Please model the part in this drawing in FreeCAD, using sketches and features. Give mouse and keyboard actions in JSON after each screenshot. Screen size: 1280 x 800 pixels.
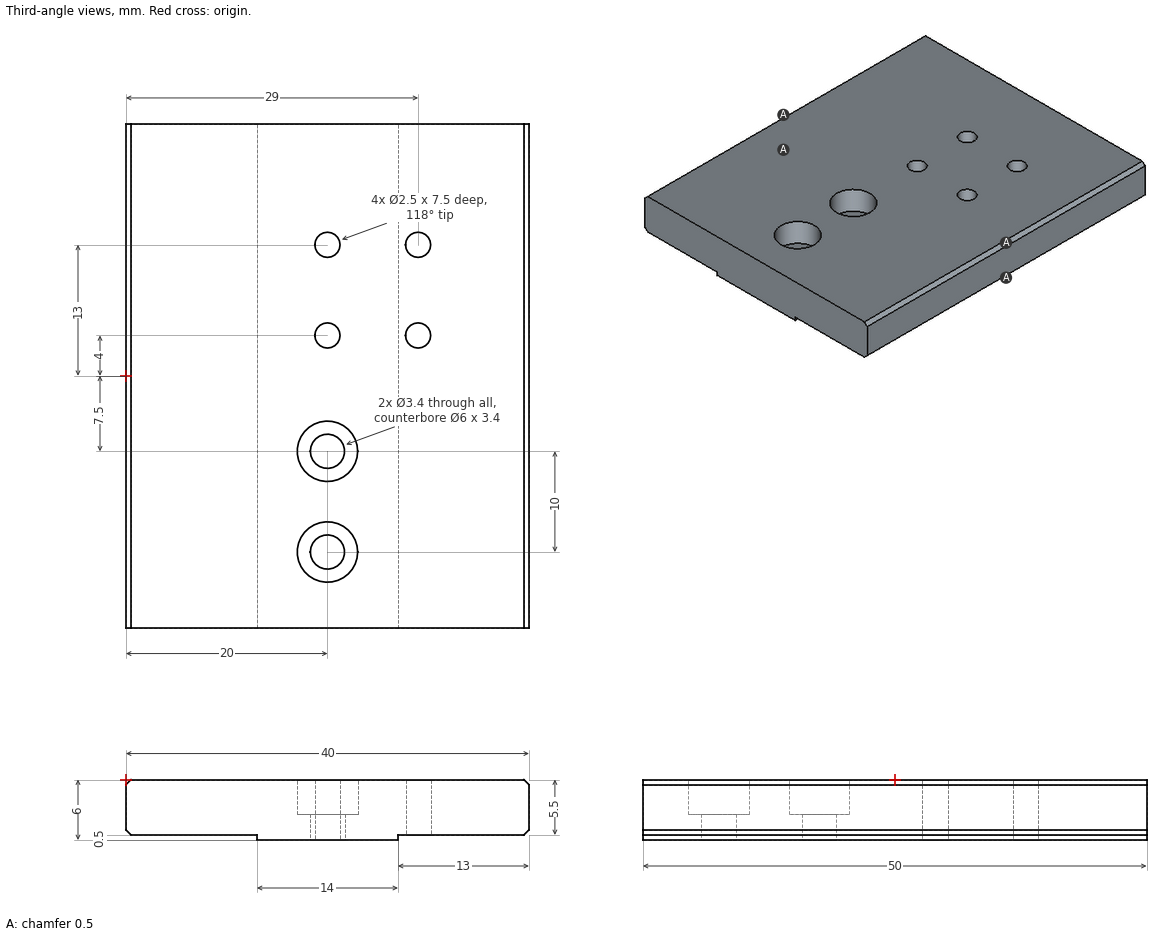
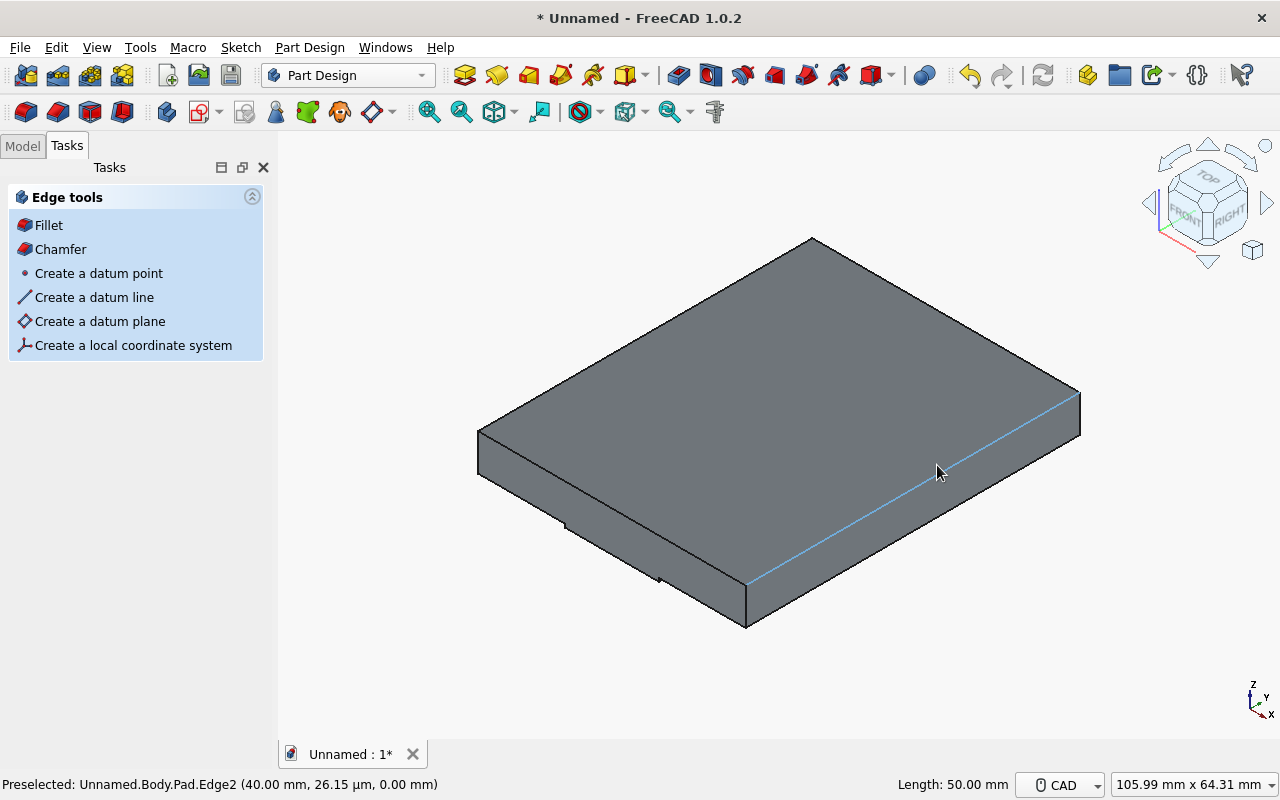
{"action": "key", "text": "2"}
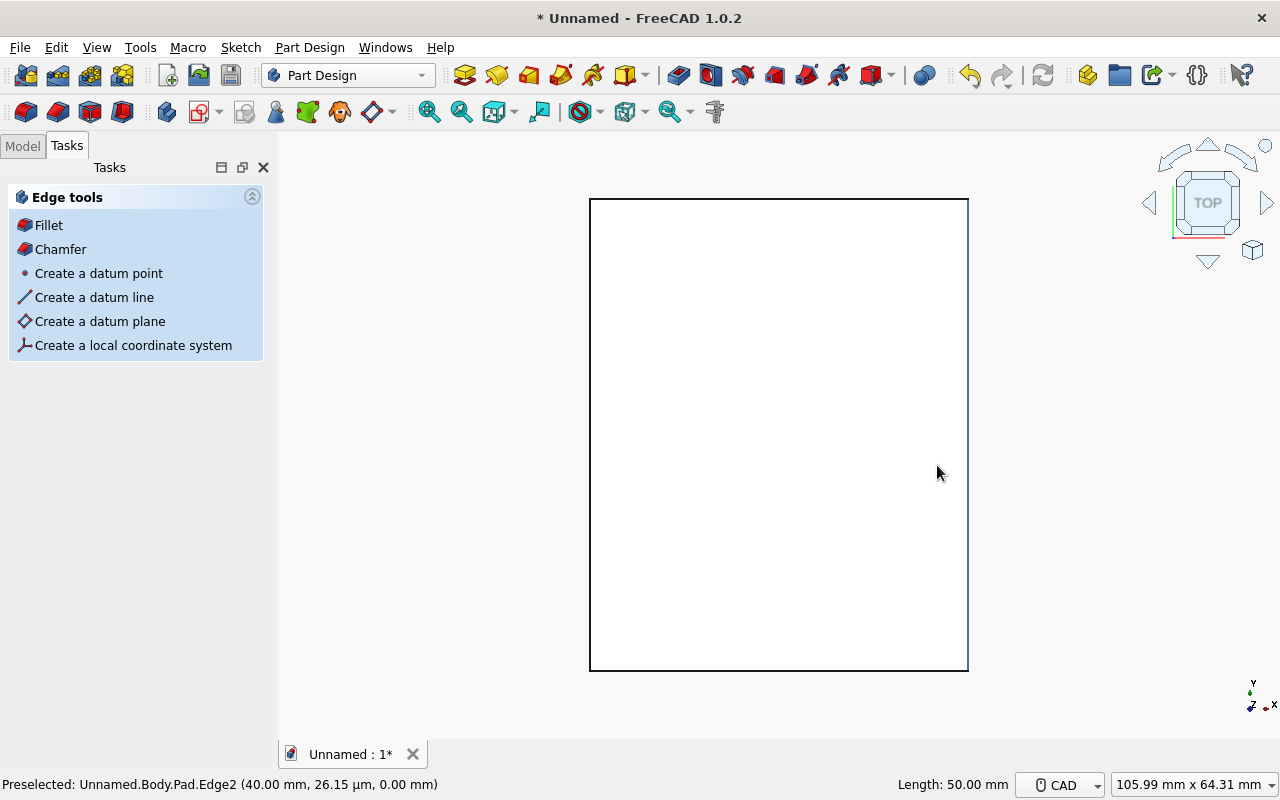
{"action": "key", "text": "1"}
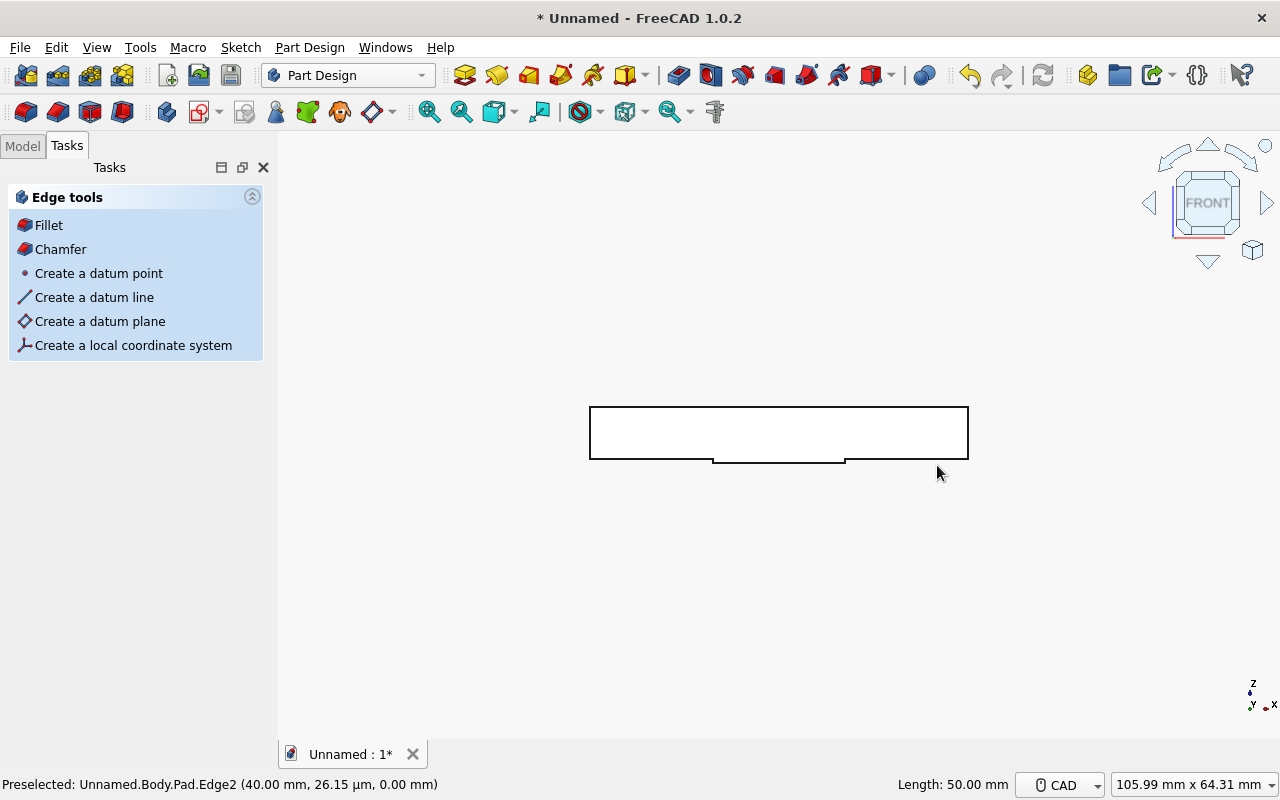
{"action": "left_click", "coordinate": [430, 112]}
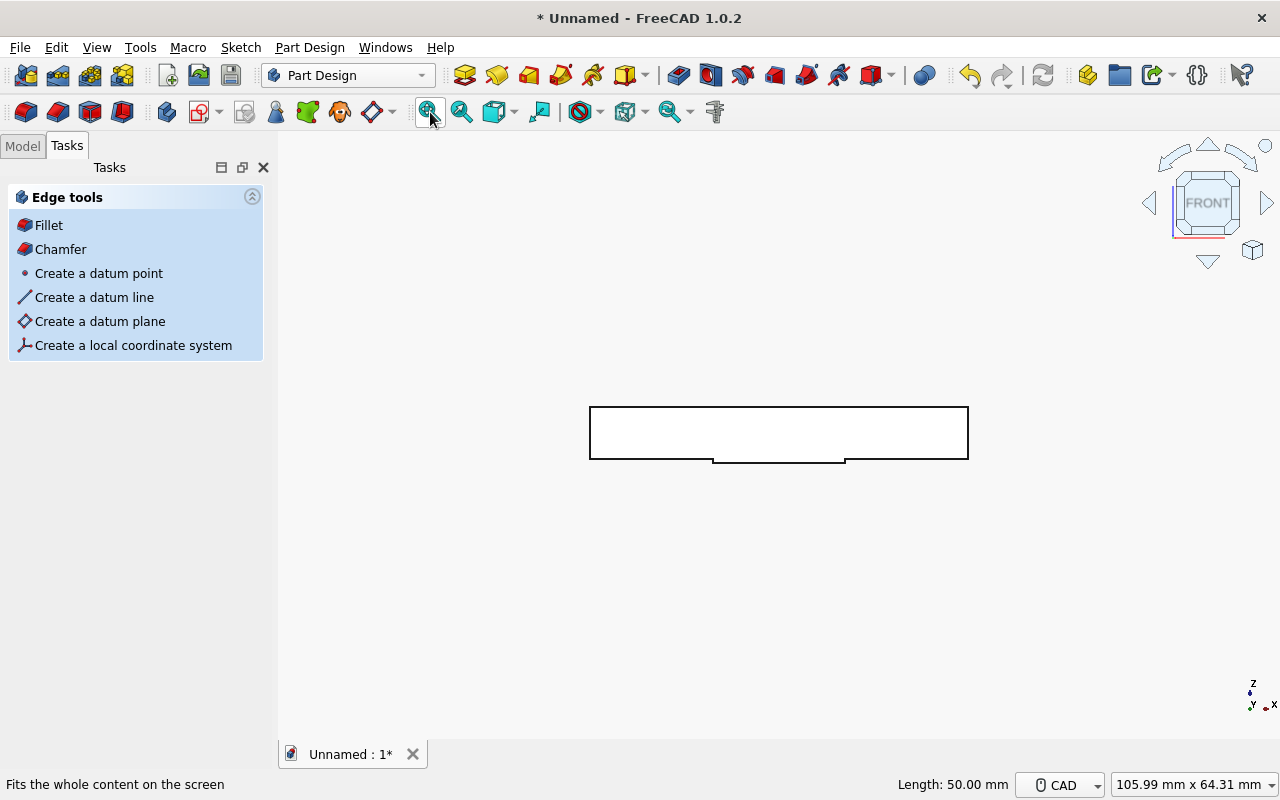
{"action": "key", "text": "3"}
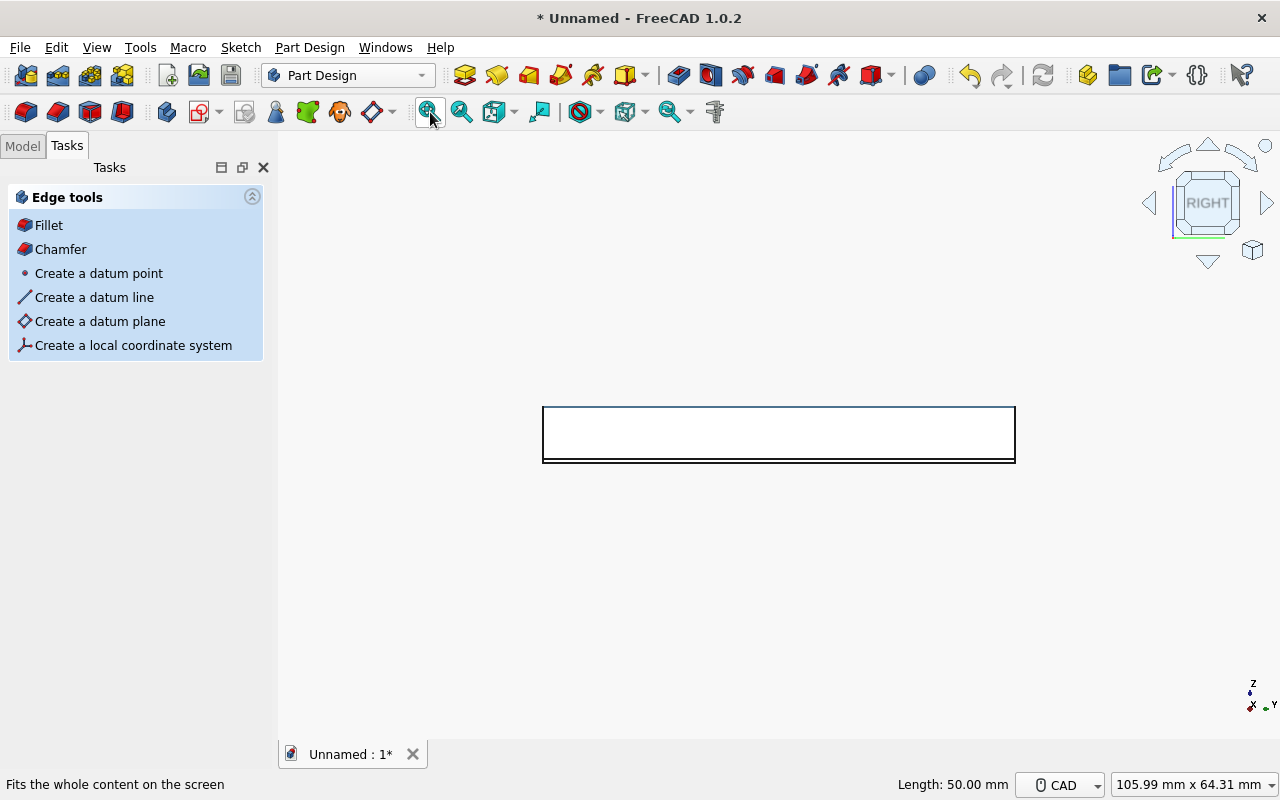
{"action": "left_click", "coordinate": [779, 458], "text": "ctrl"}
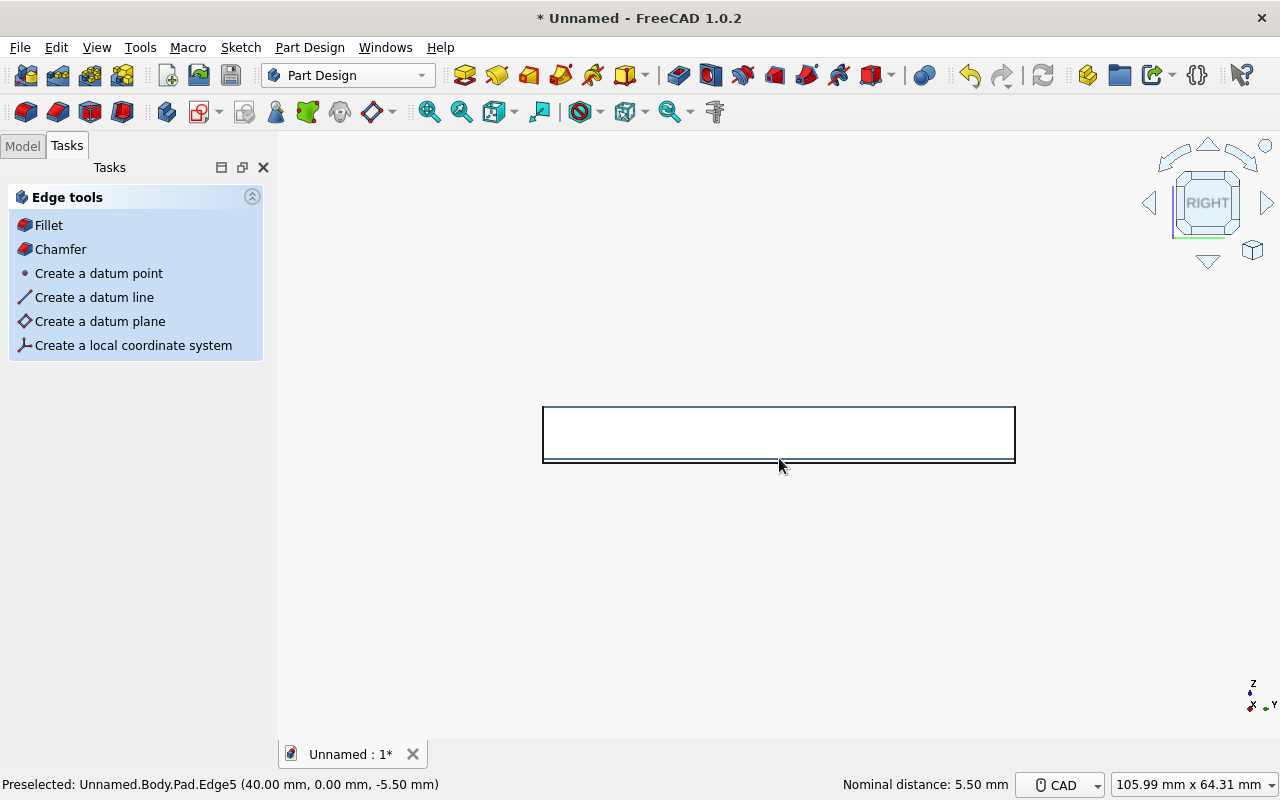
{"action": "key", "text": "5"}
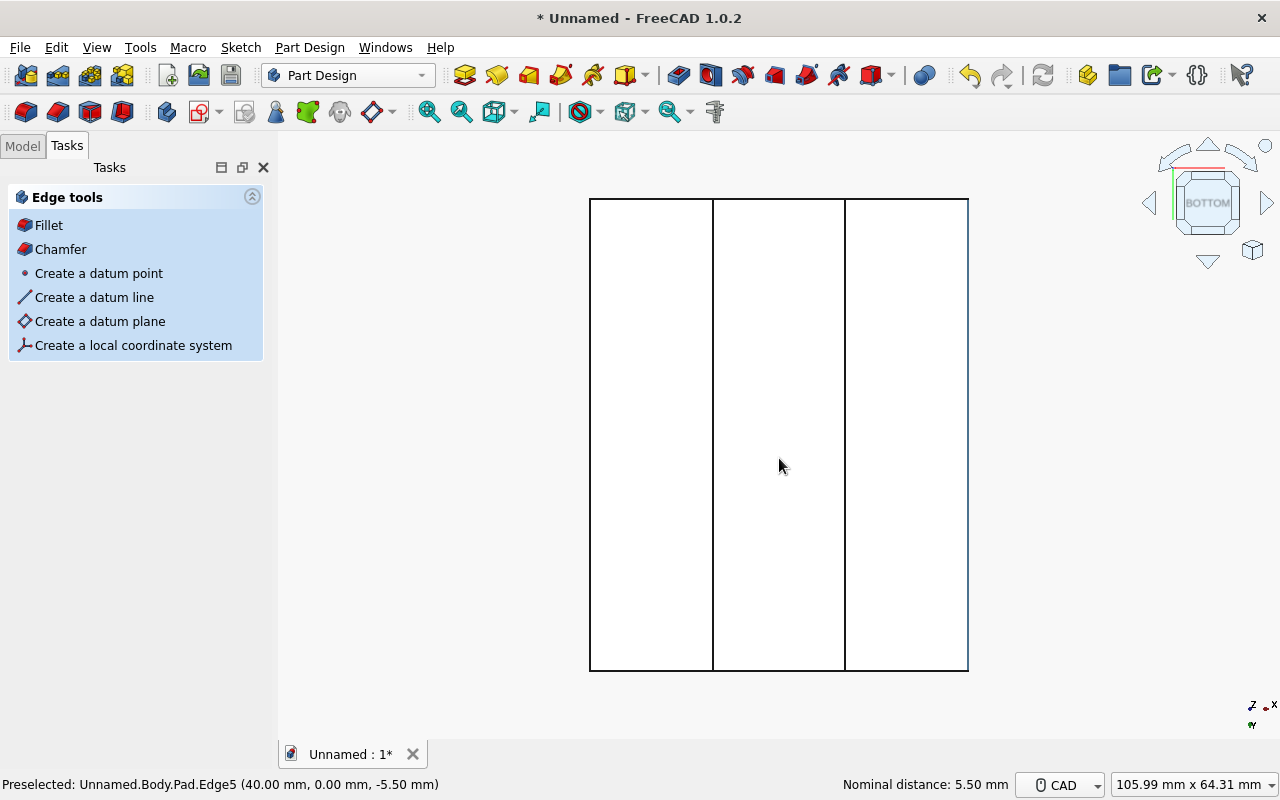
{"action": "left_click", "coordinate": [590, 434], "text": "ctrl"}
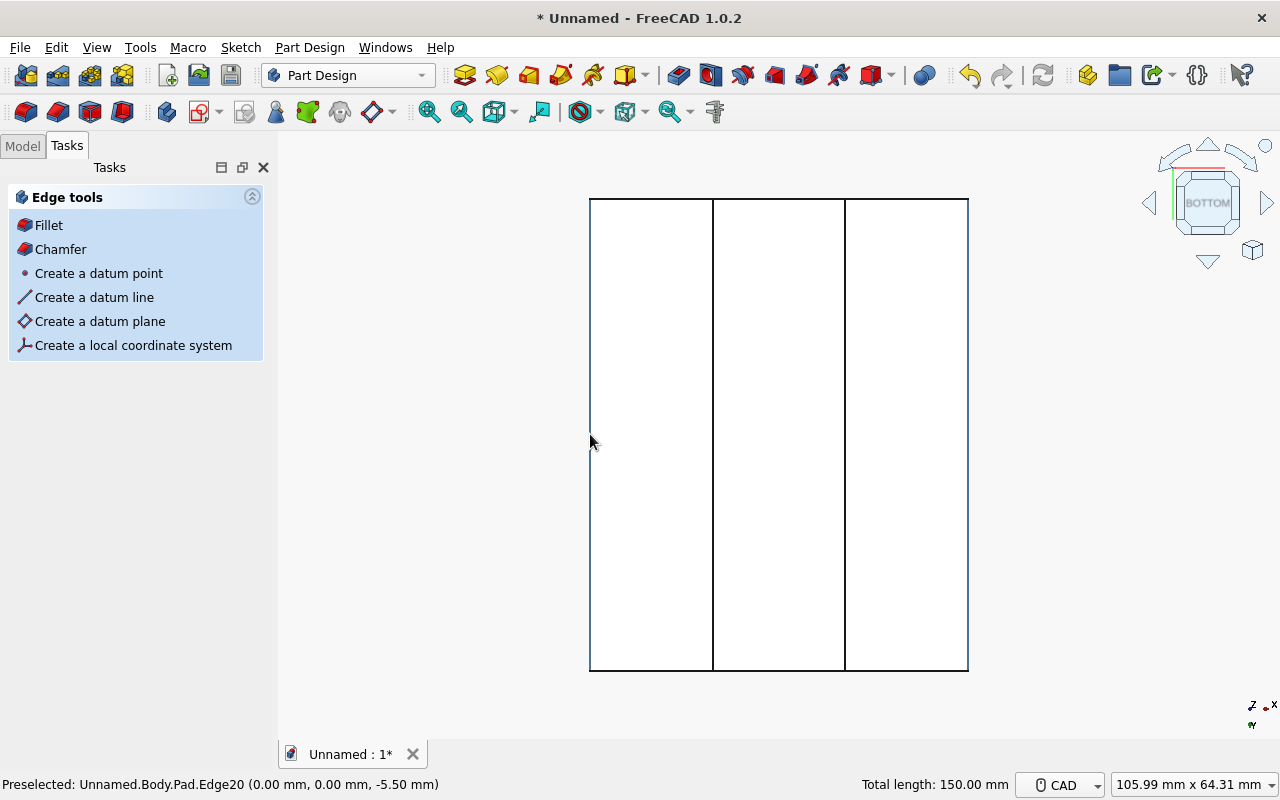
{"action": "key", "text": "4"}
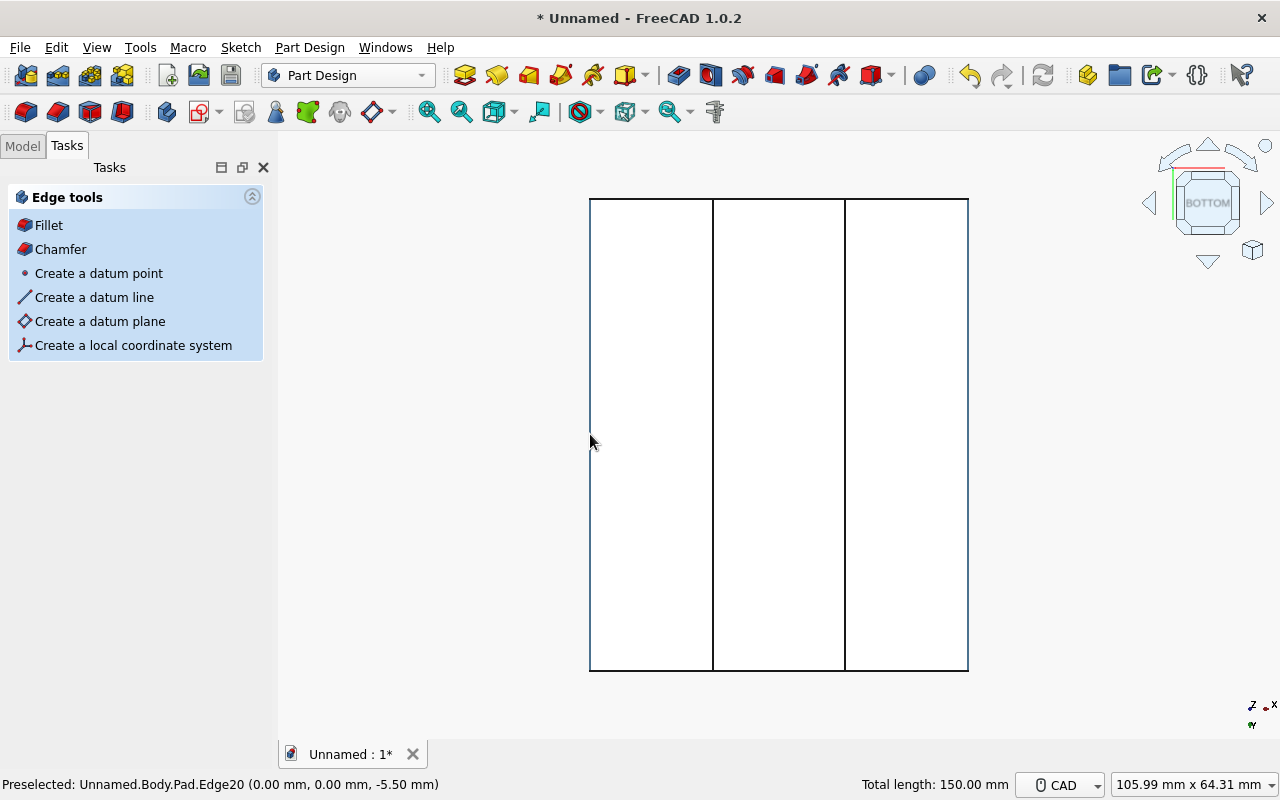
{"action": "left_click", "coordinate": [430, 112]}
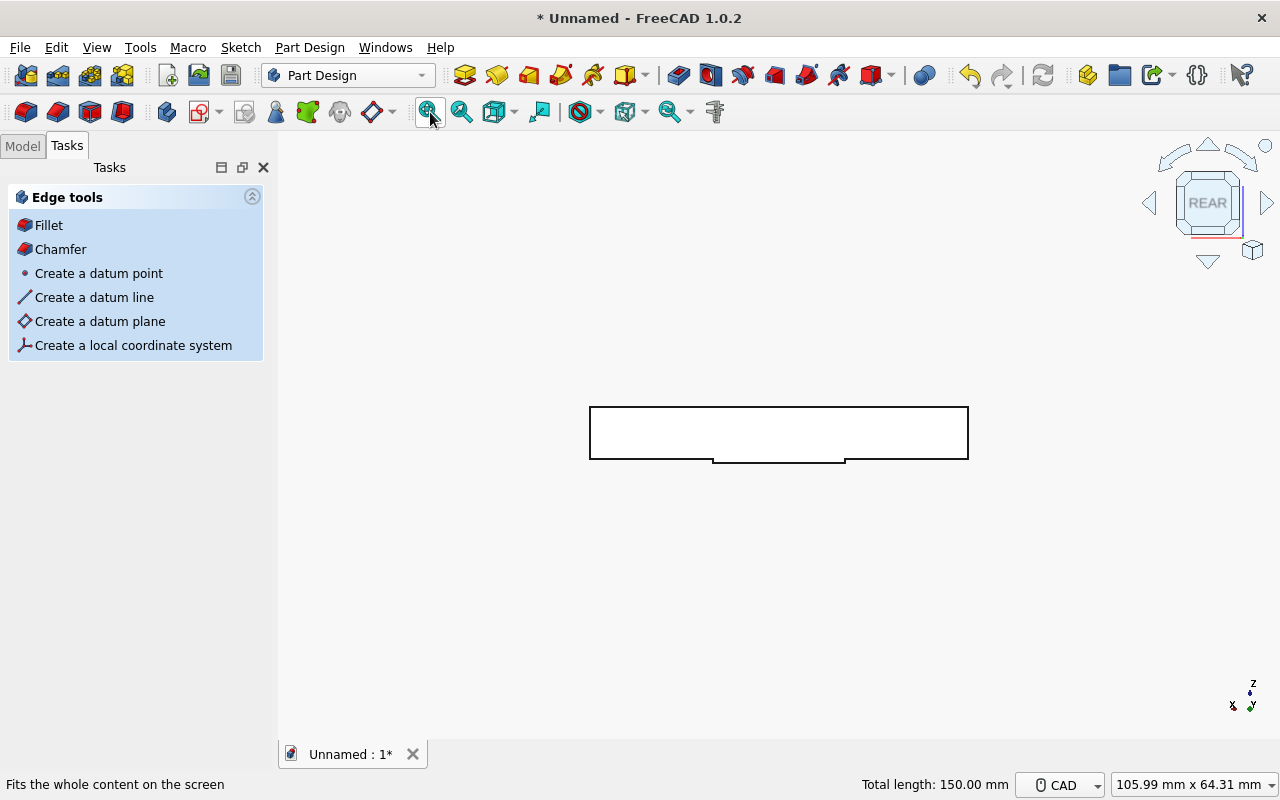
{"action": "key", "text": "6"}